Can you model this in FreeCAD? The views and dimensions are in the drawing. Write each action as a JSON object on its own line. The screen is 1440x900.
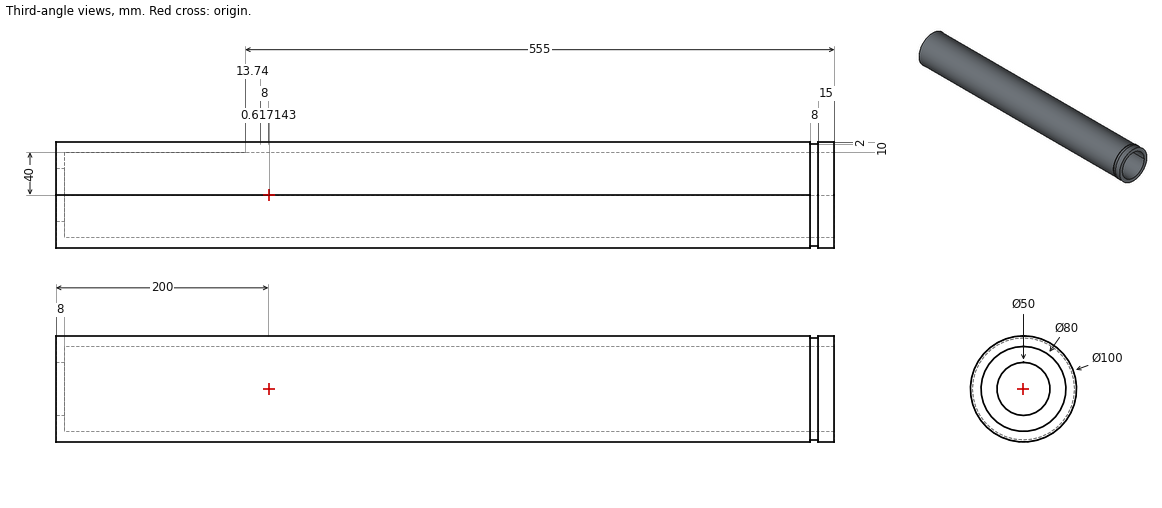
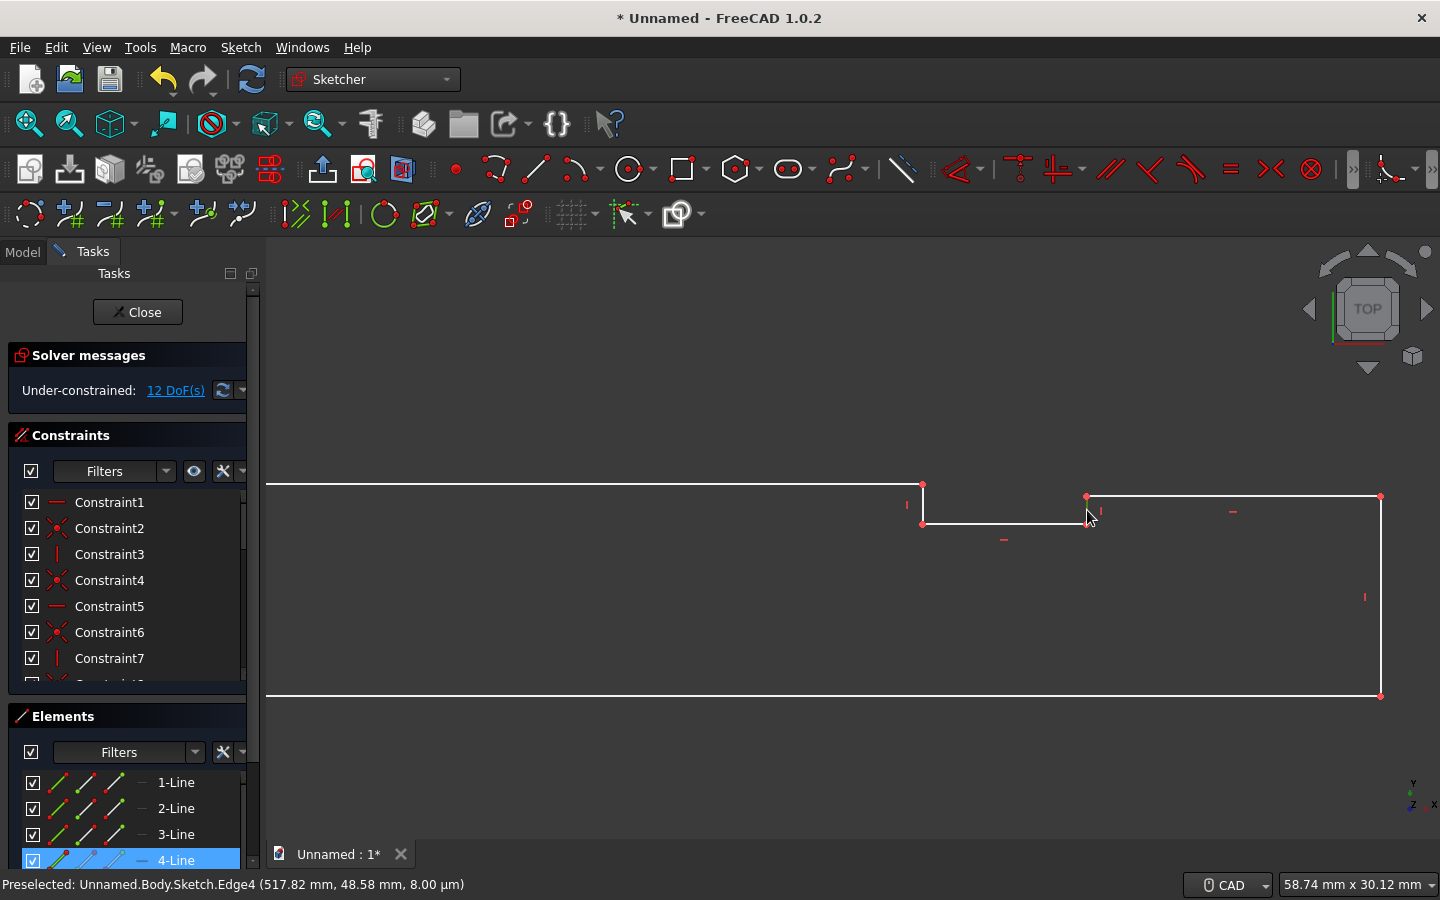
{"action": "left_click", "coordinate": [982, 170]}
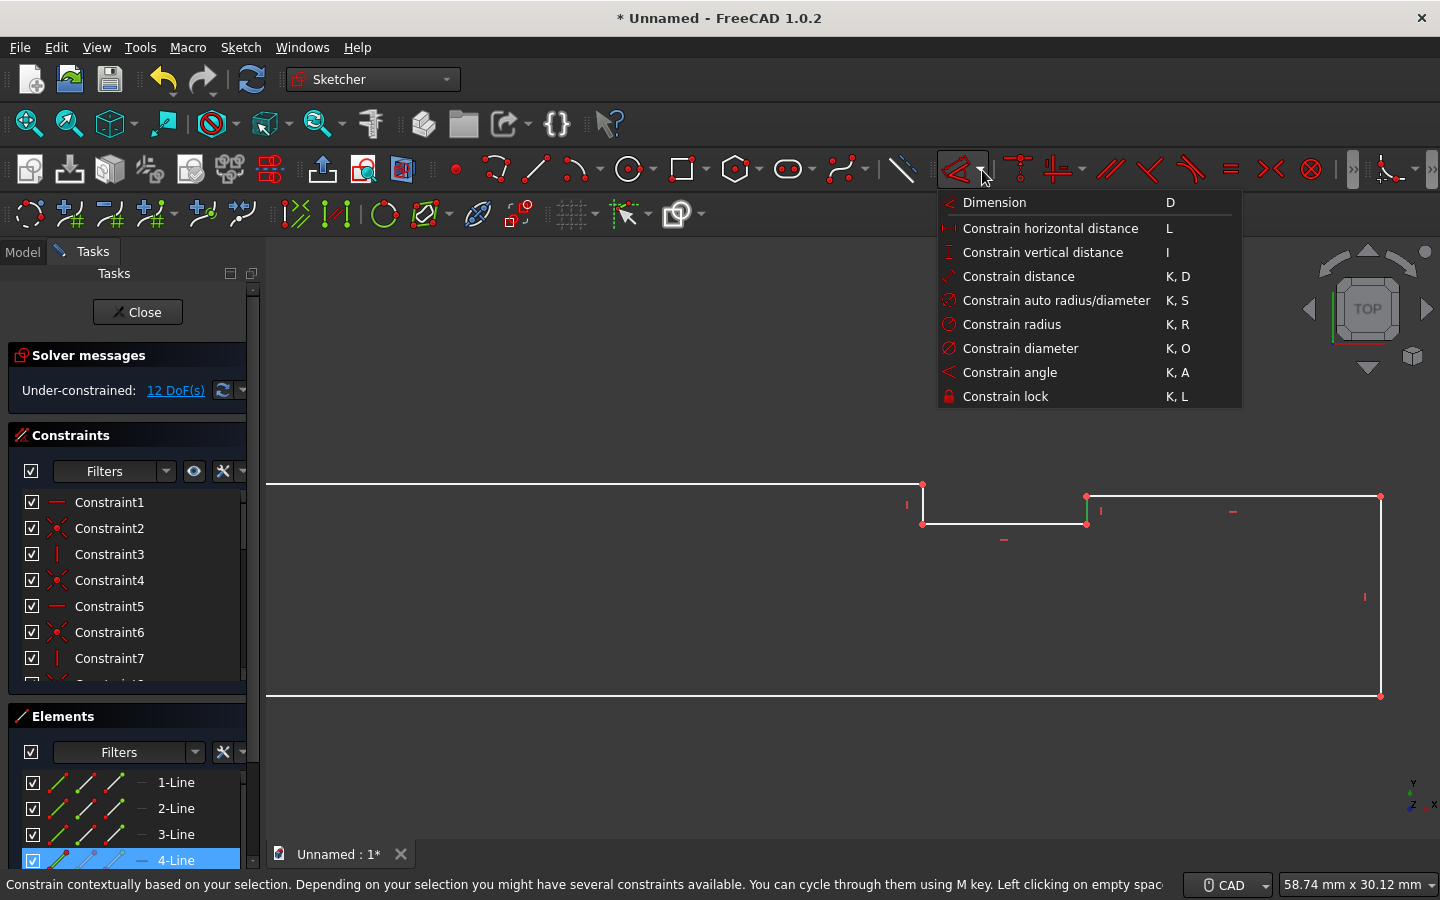
{"action": "left_click", "coordinate": [1090, 252]}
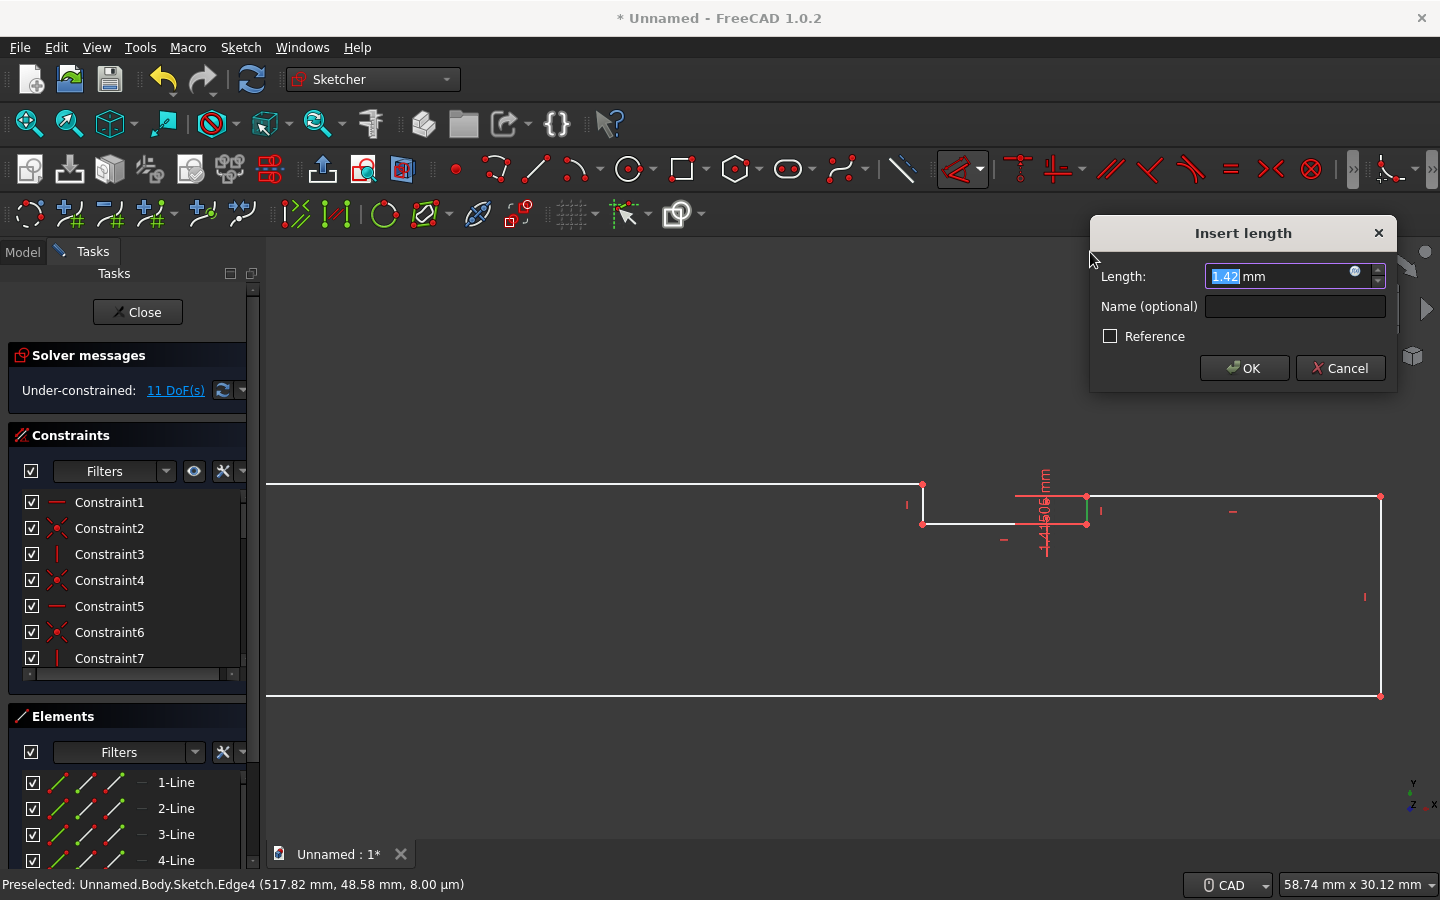
{"action": "type", "text": "2"}
{"action": "key", "text": "Return"}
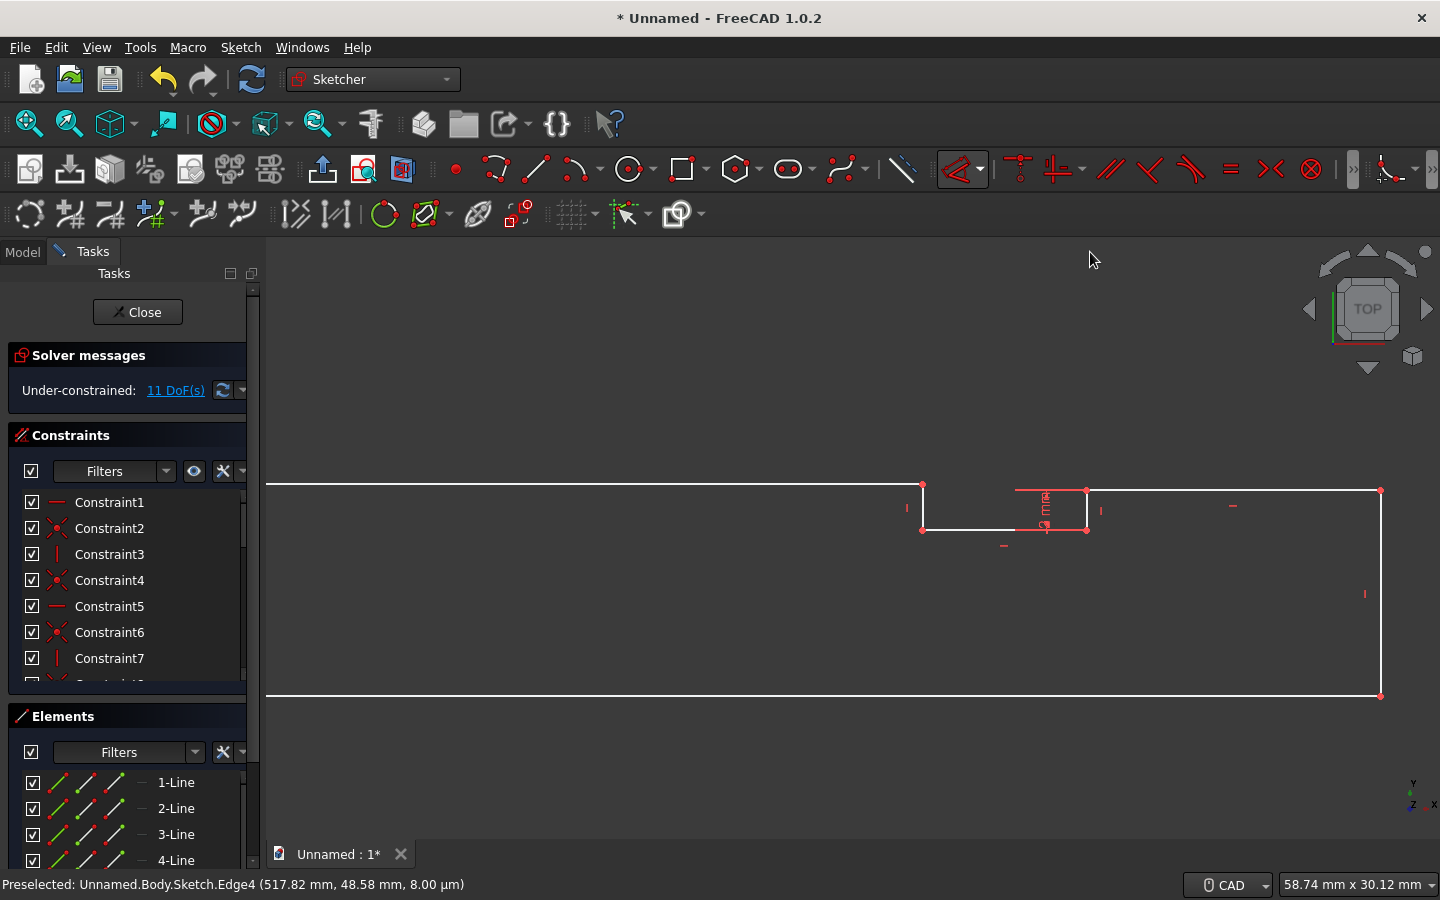
{"action": "scroll", "coordinate": [1105, 509], "scroll_direction": "down", "scroll_amount": 14}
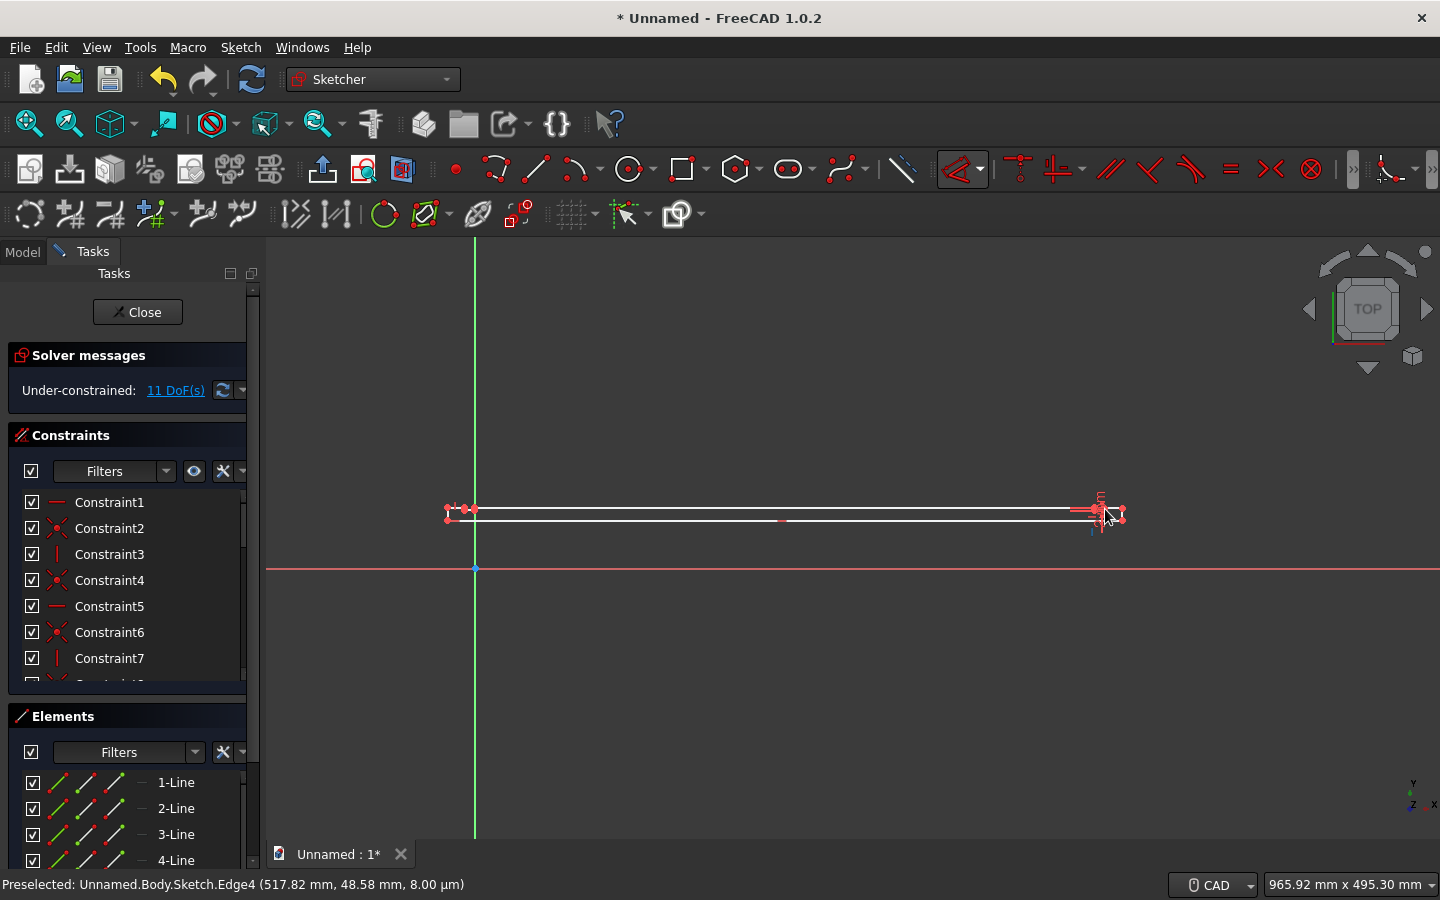
{"action": "scroll", "coordinate": [1102, 511], "scroll_direction": "up", "scroll_amount": 8}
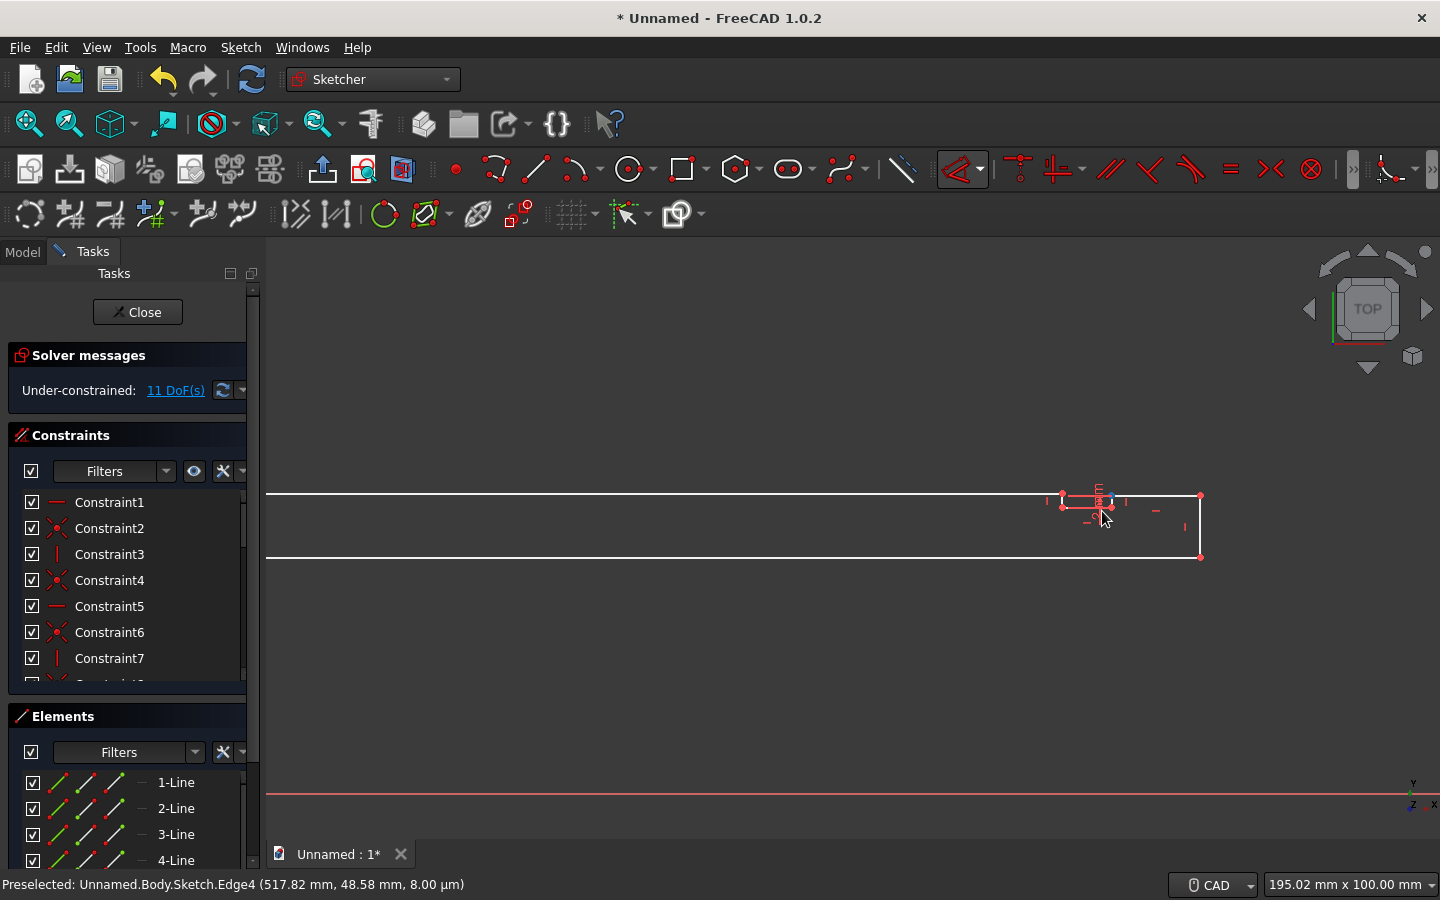
{"action": "left_click", "coordinate": [1077, 508]}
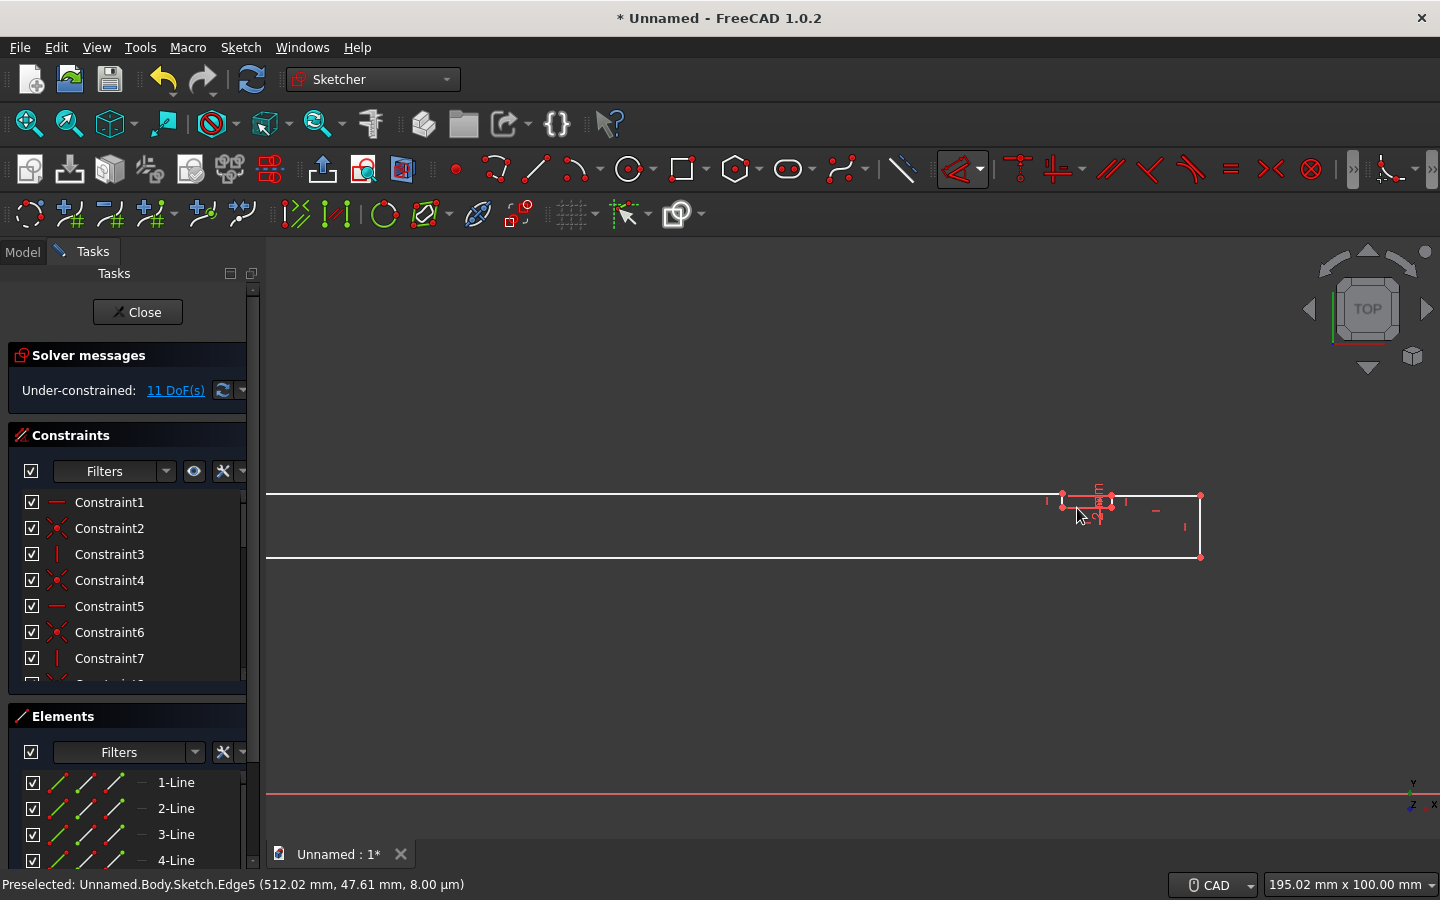
{"action": "key", "text": "l"}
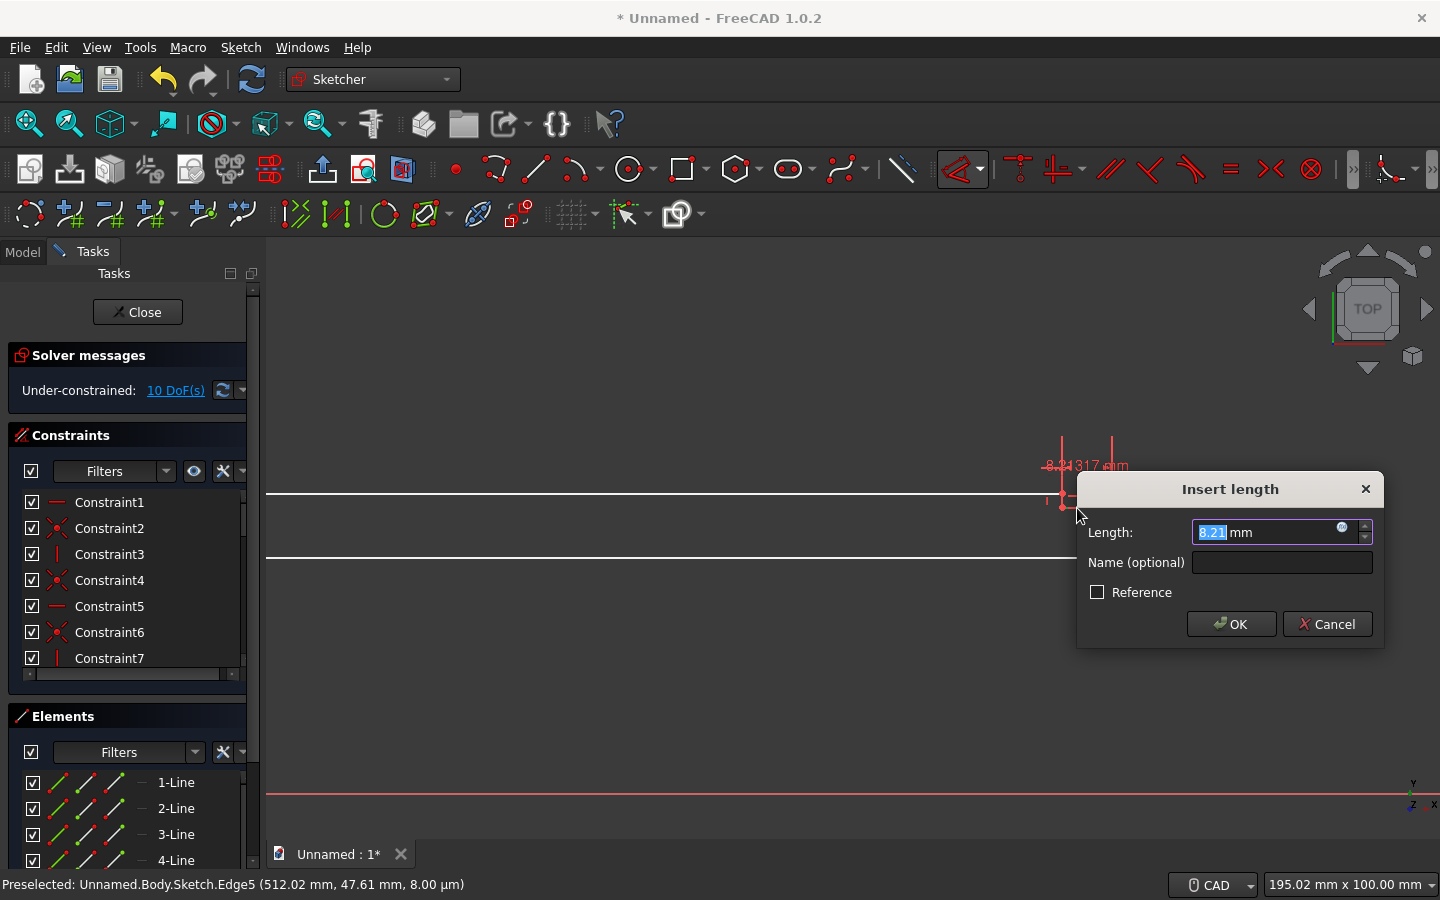
{"action": "type", "text": "8"}
{"action": "key", "text": "Return"}